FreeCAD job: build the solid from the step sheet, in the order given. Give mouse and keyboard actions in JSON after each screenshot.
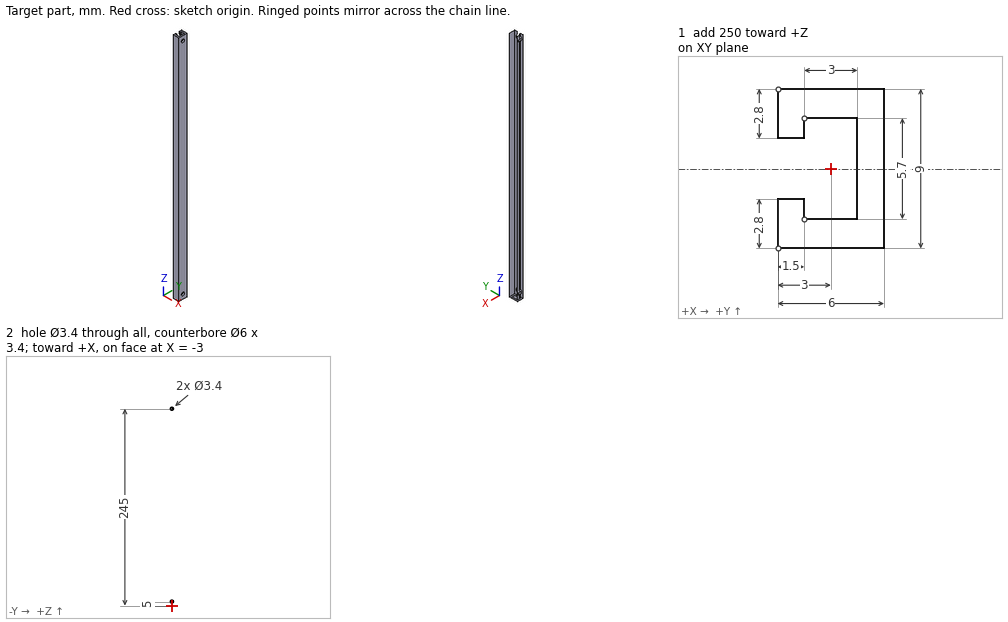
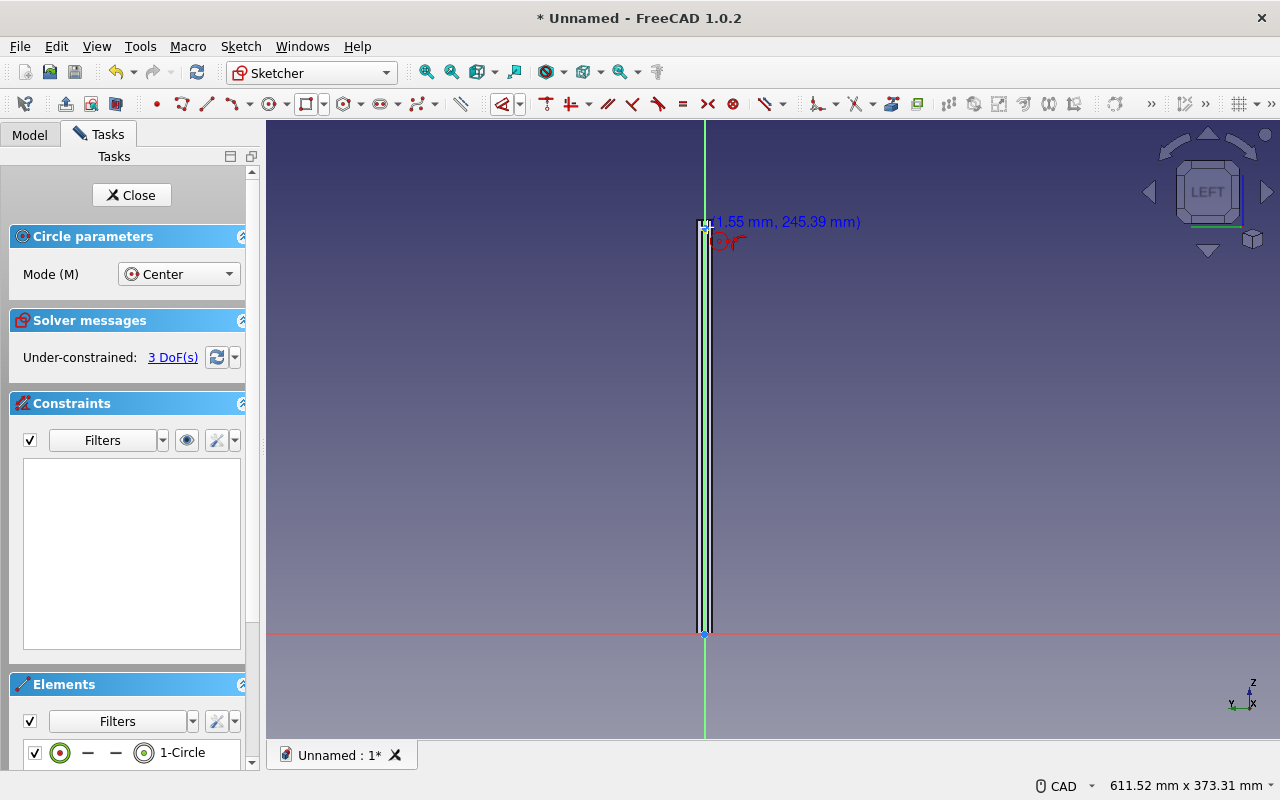
{"action": "scroll", "coordinate": [705, 626], "scroll_direction": "up", "scroll_amount": 11}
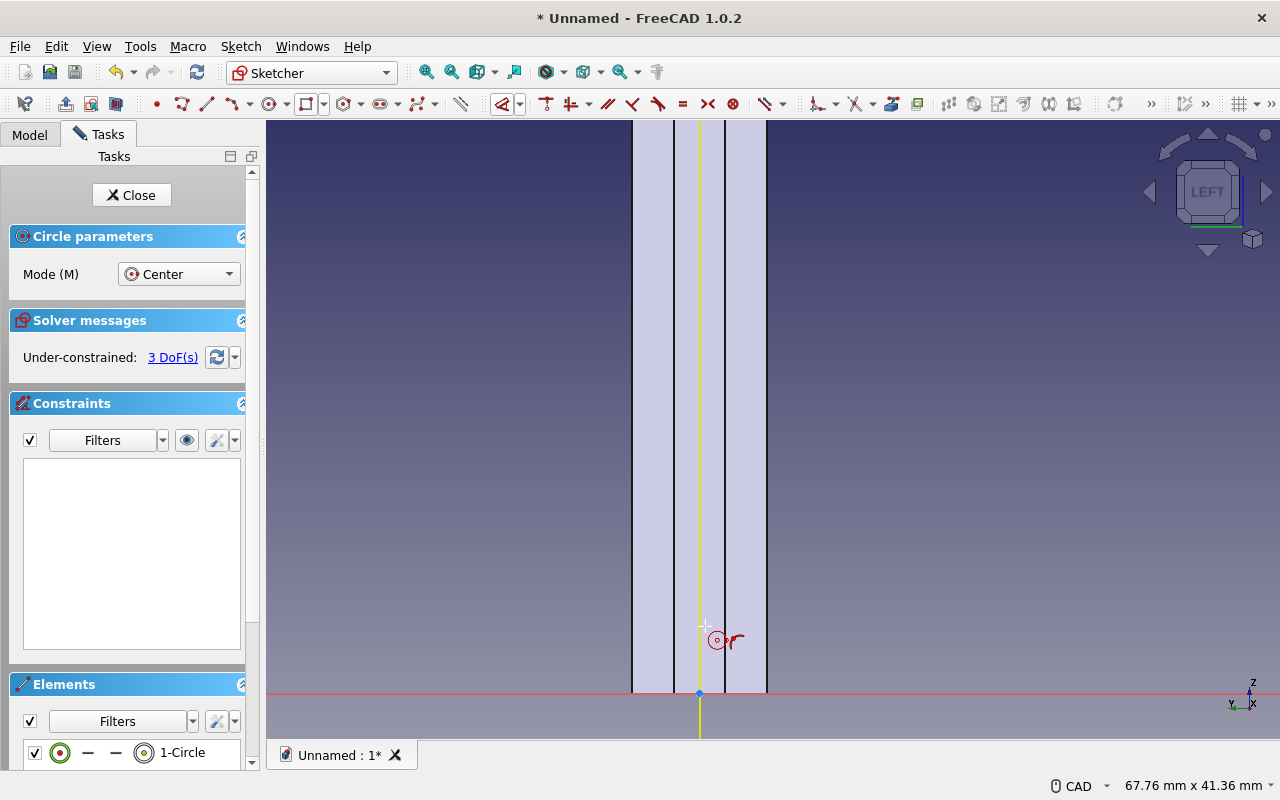
{"action": "scroll", "coordinate": [705, 627], "scroll_direction": "down", "scroll_amount": 11}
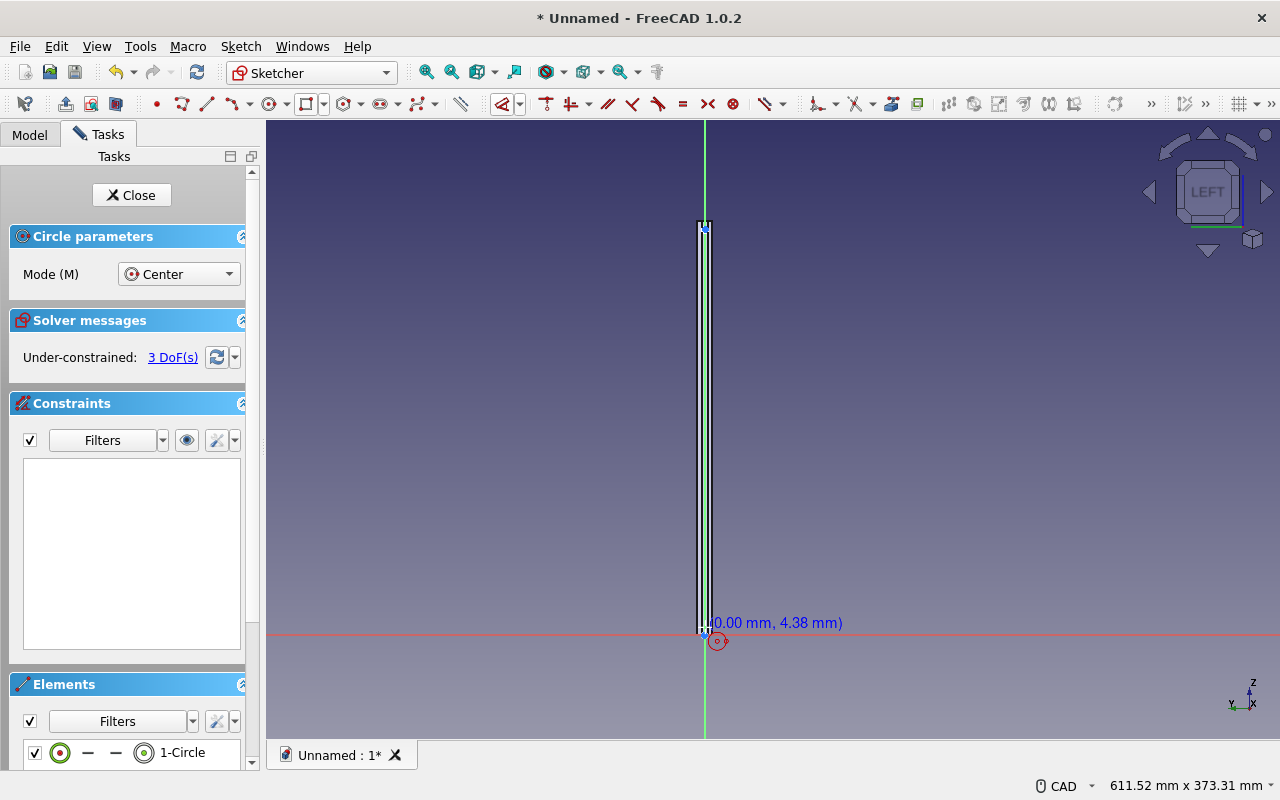
{"action": "scroll", "coordinate": [705, 627], "scroll_direction": "up", "scroll_amount": 4}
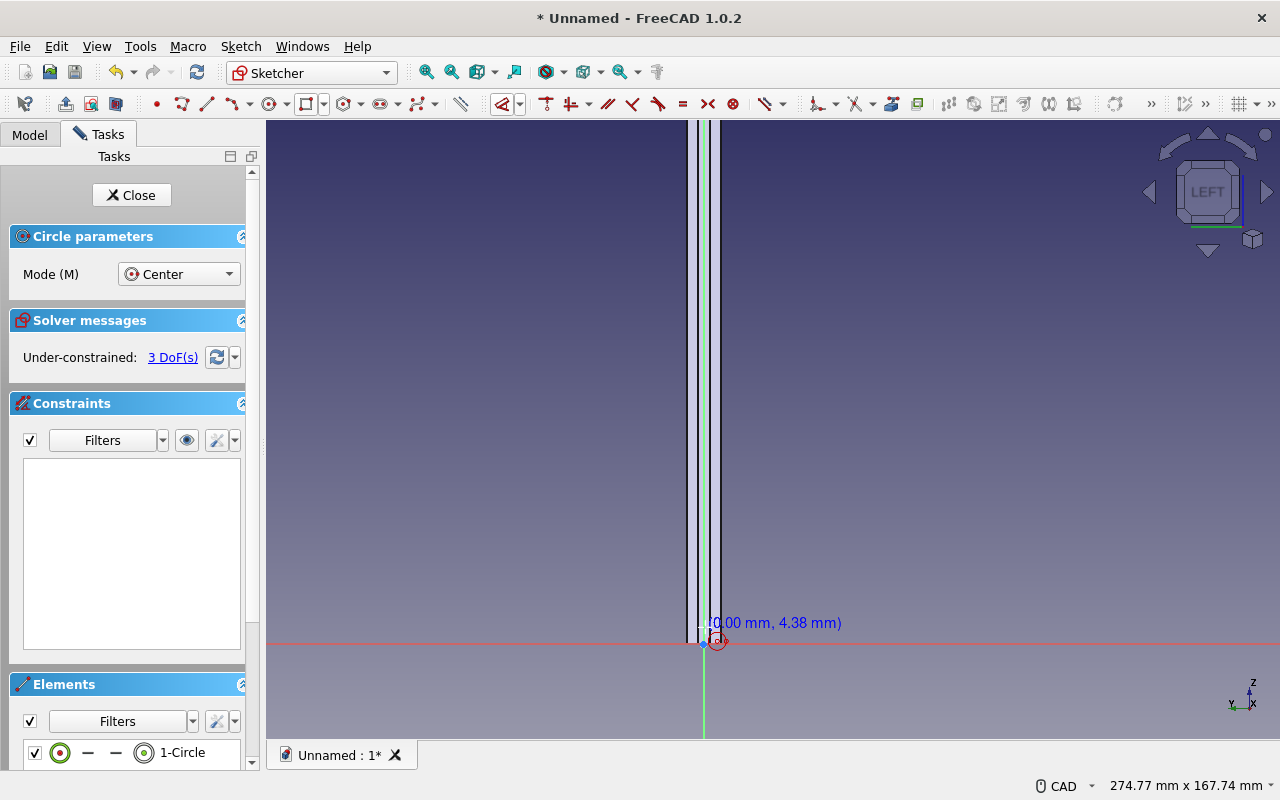
{"action": "left_click", "coordinate": [704, 626]}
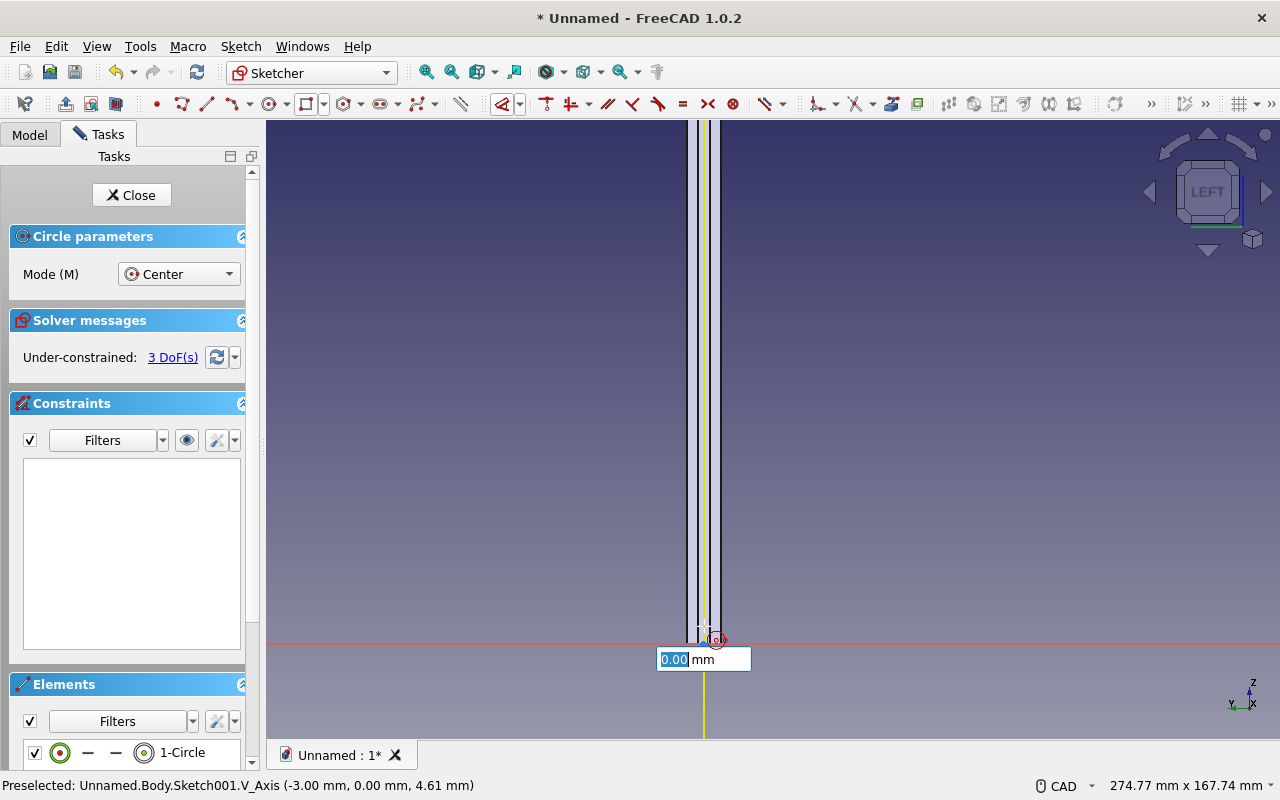
{"action": "scroll", "coordinate": [710, 623], "scroll_direction": "up", "scroll_amount": 5}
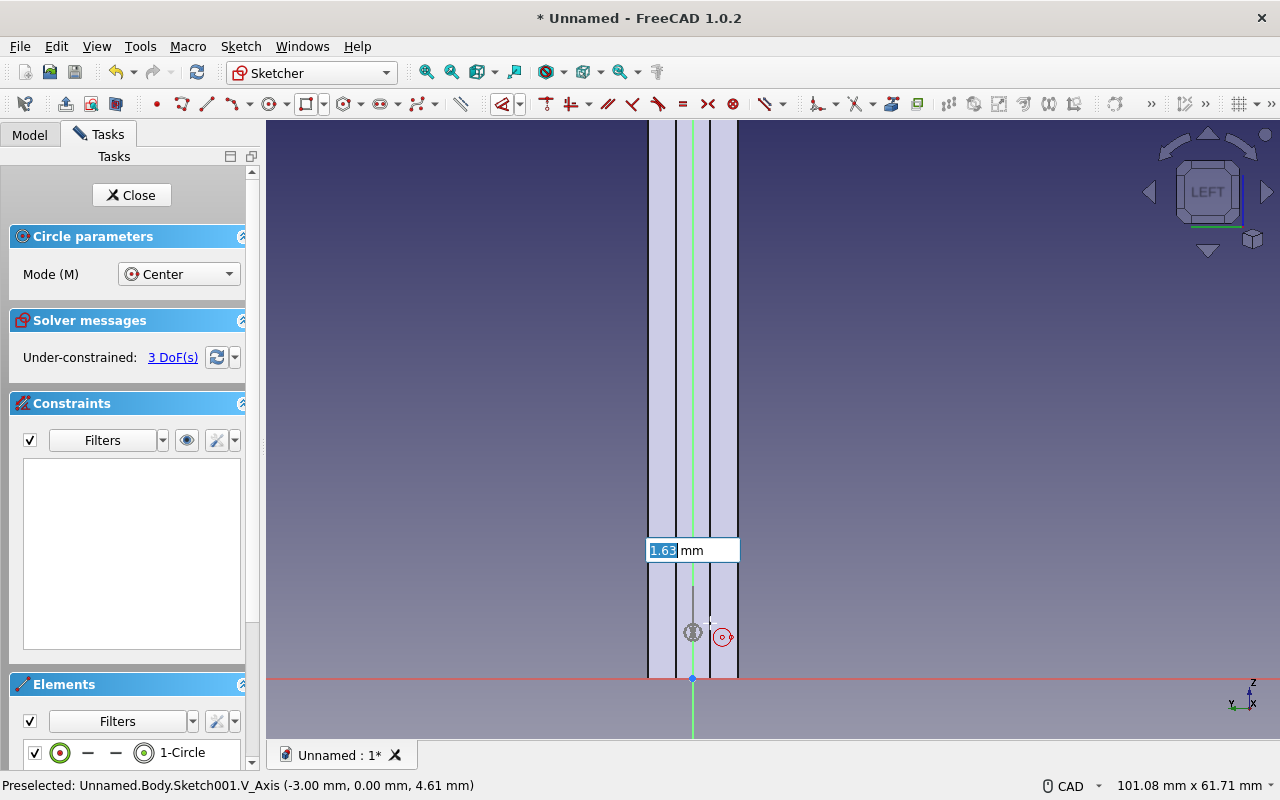
{"action": "left_click", "coordinate": [709, 623]}
{"action": "key", "text": "Escape"}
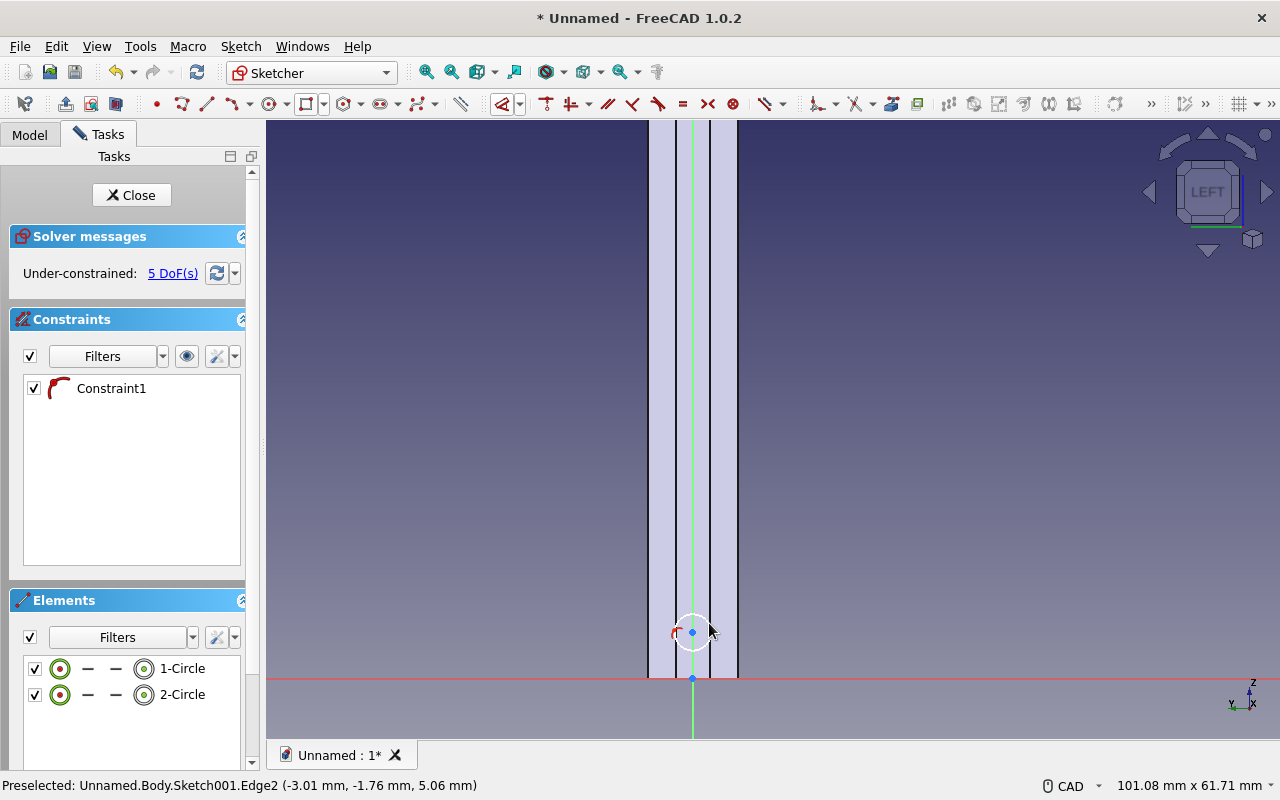
{"action": "scroll", "coordinate": [707, 625], "scroll_direction": "down", "scroll_amount": 9}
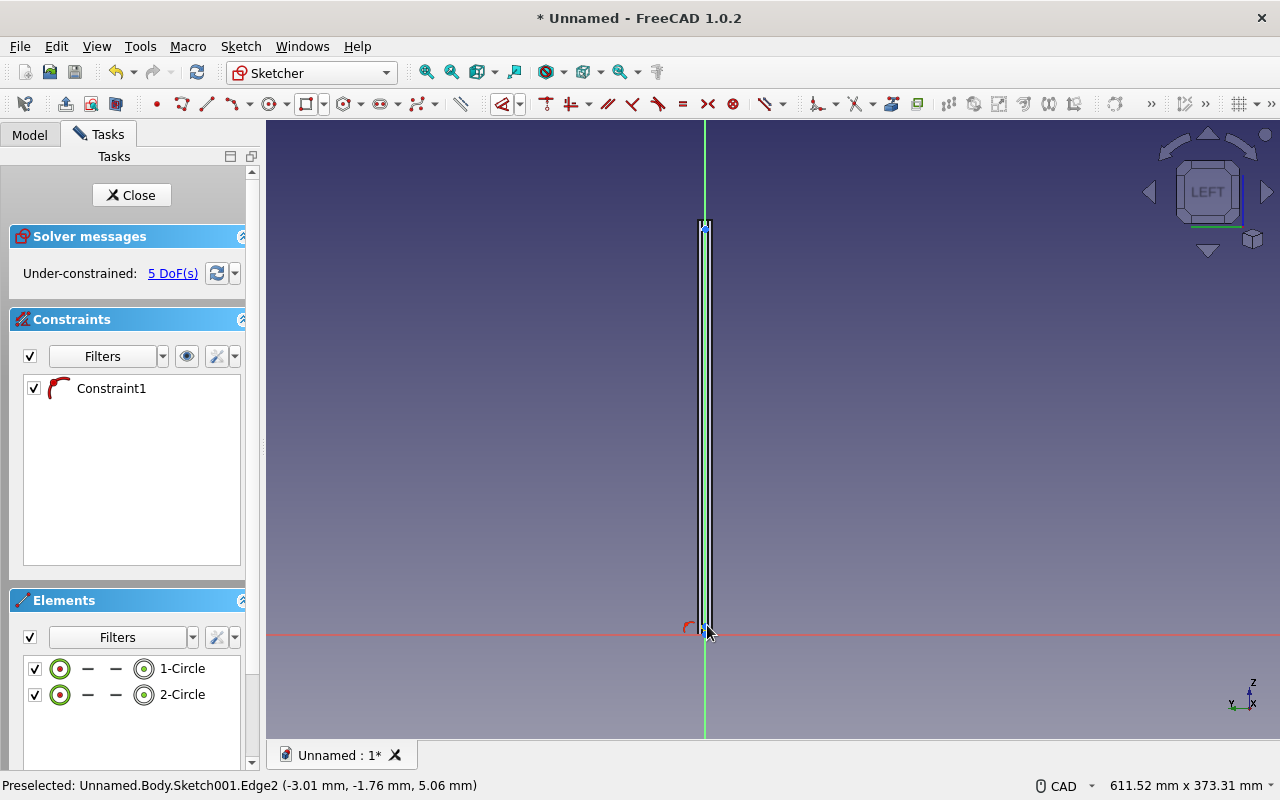
{"action": "scroll", "coordinate": [707, 227], "scroll_direction": "up", "scroll_amount": 9}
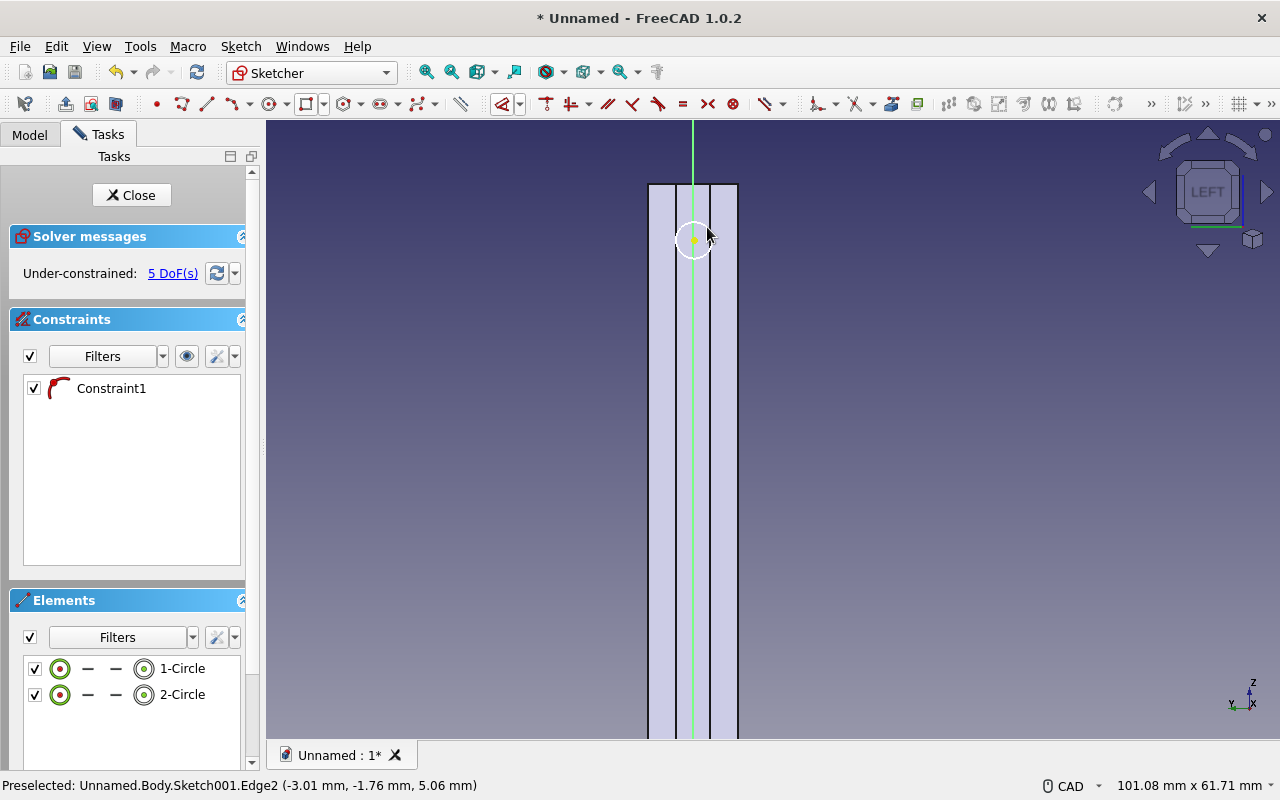
{"action": "left_click", "coordinate": [707, 227]}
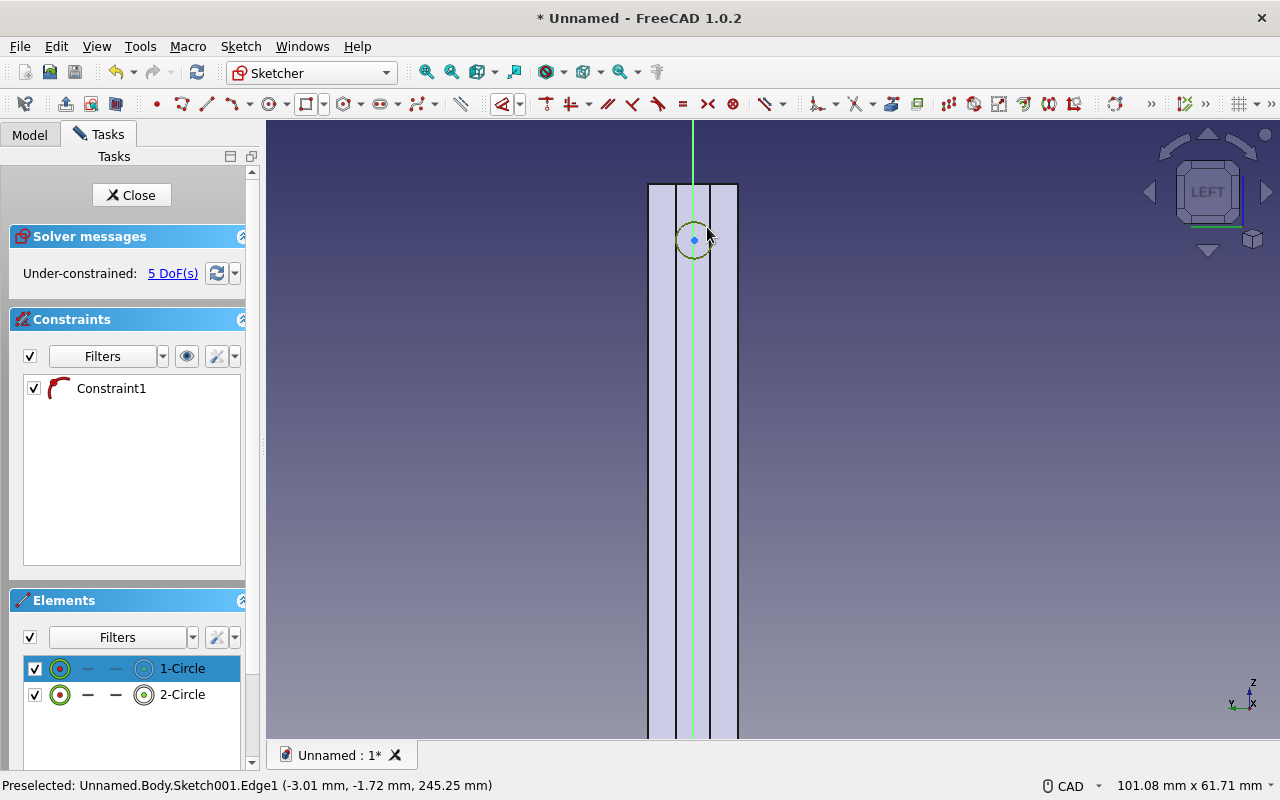
{"action": "scroll", "coordinate": [707, 227], "scroll_direction": "down", "scroll_amount": 9}